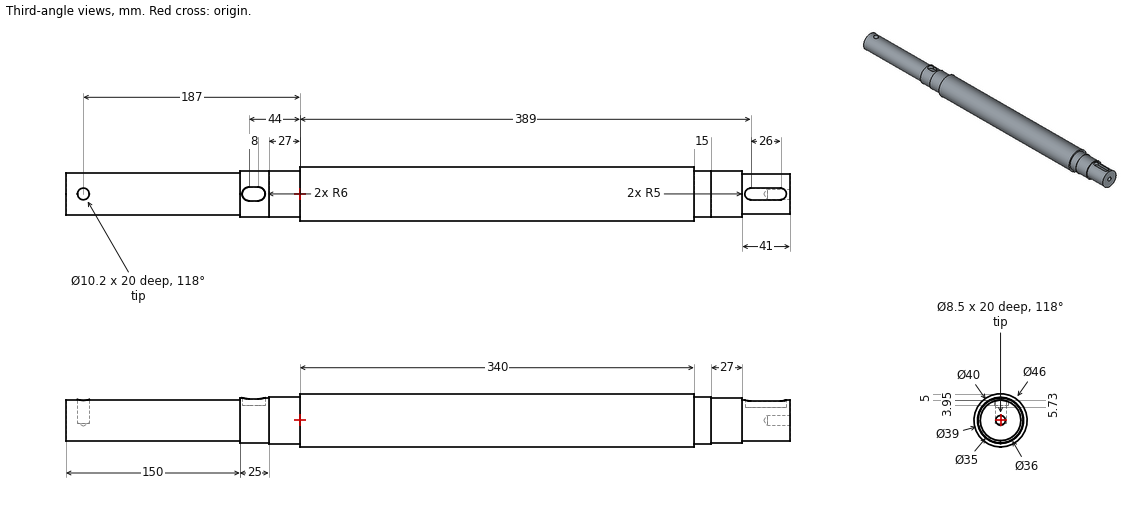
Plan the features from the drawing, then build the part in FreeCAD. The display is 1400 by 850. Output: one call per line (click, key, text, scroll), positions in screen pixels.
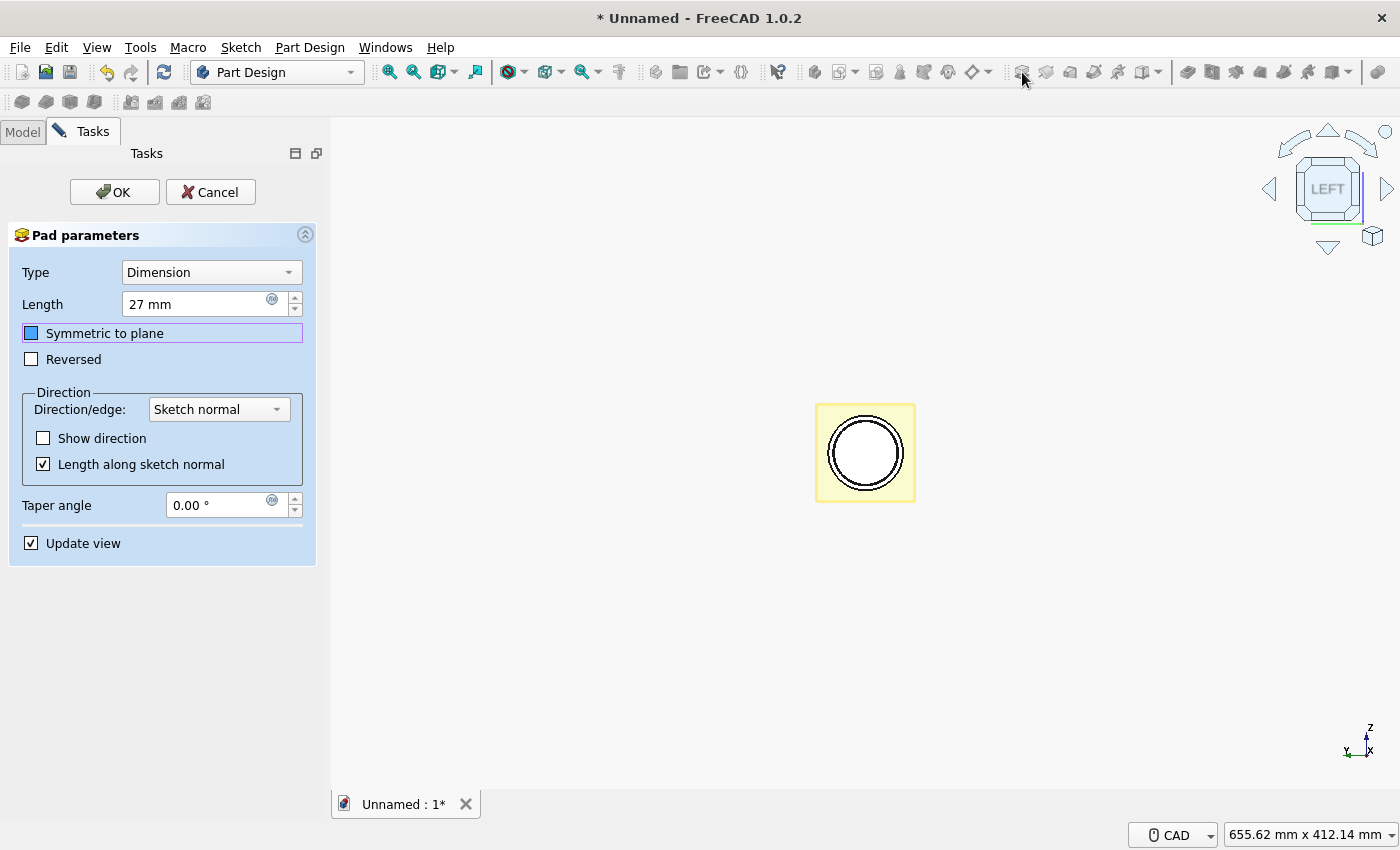
click(30, 359)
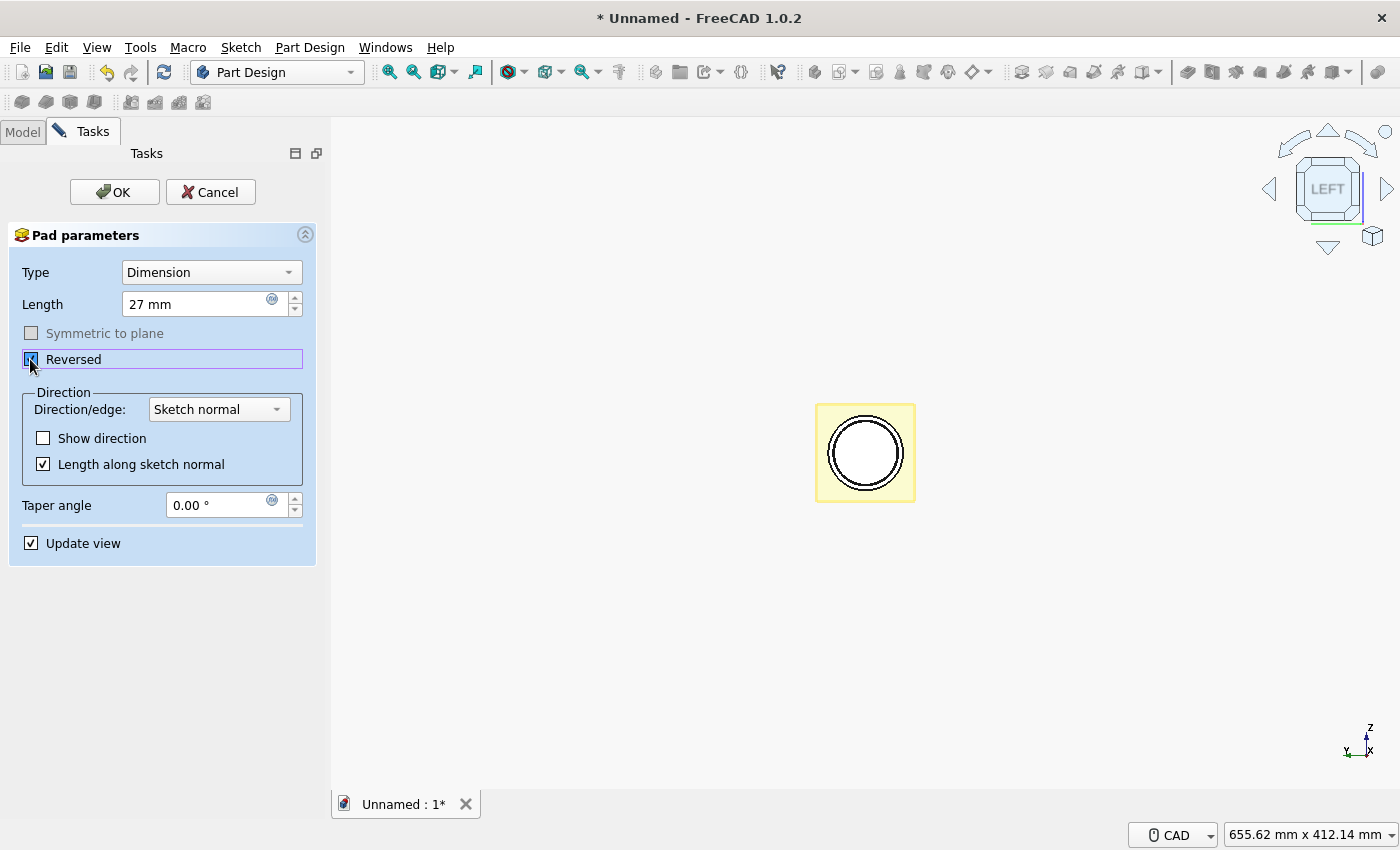
click(115, 192)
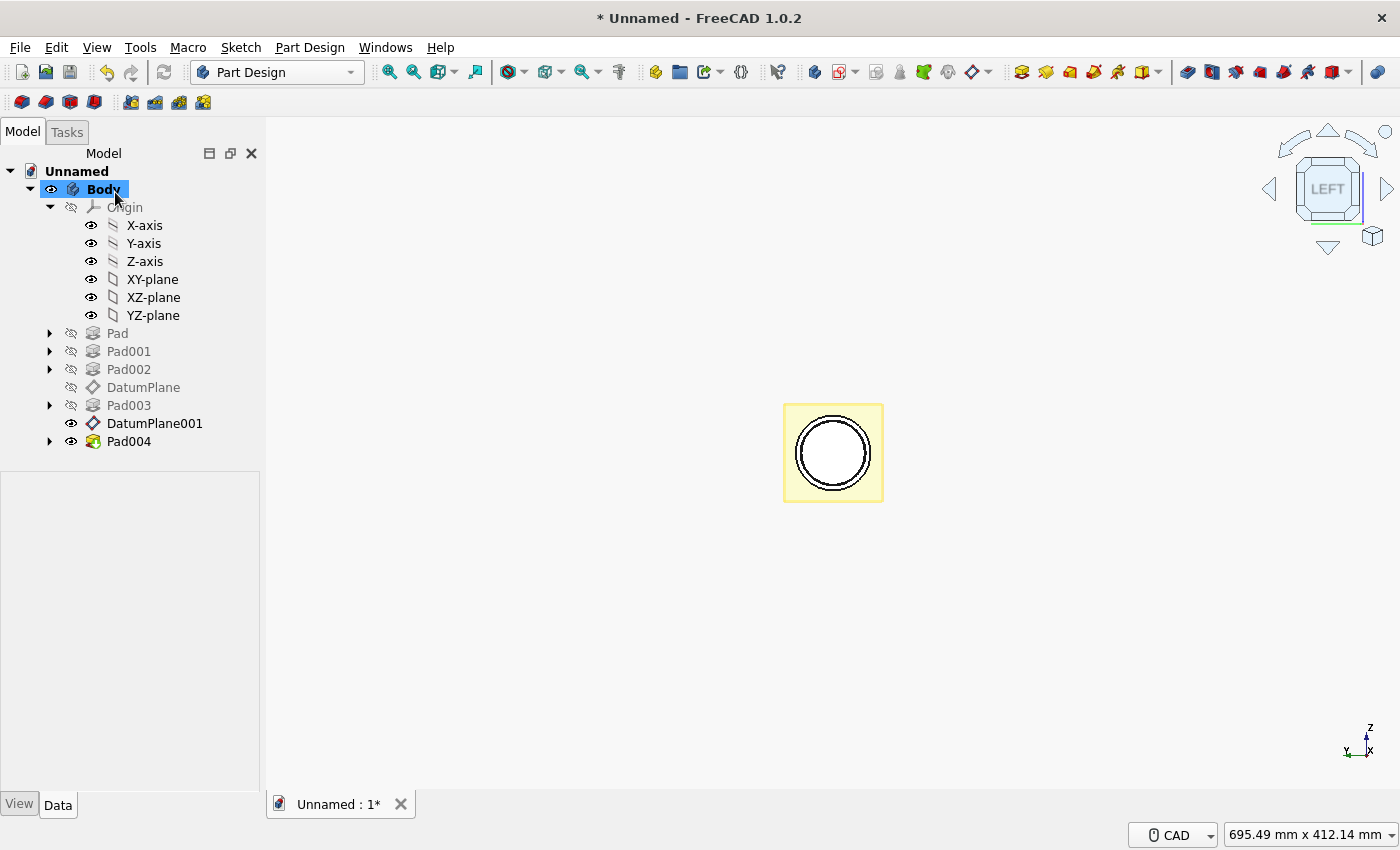
click(116, 423)
key(space)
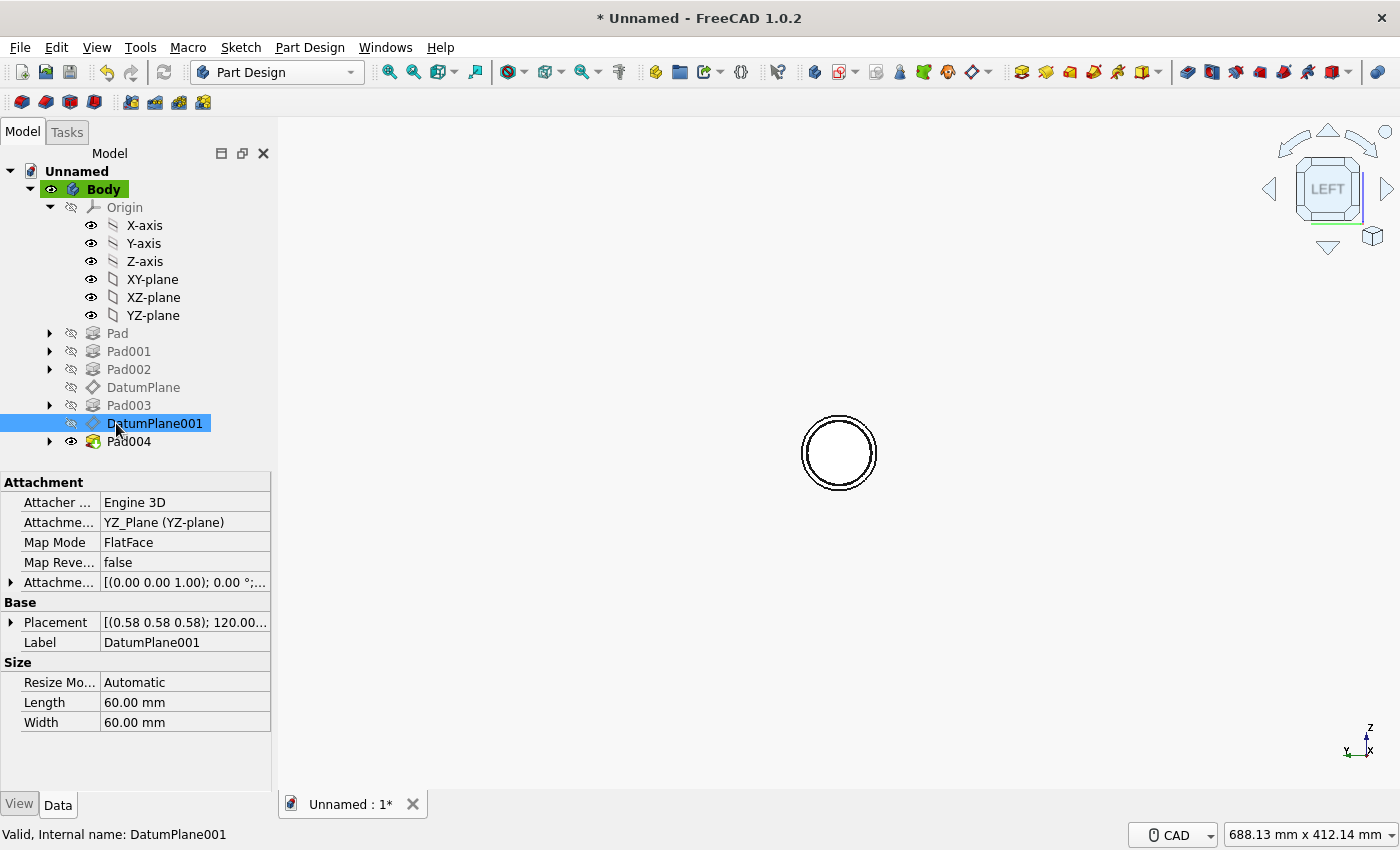
click(390, 72)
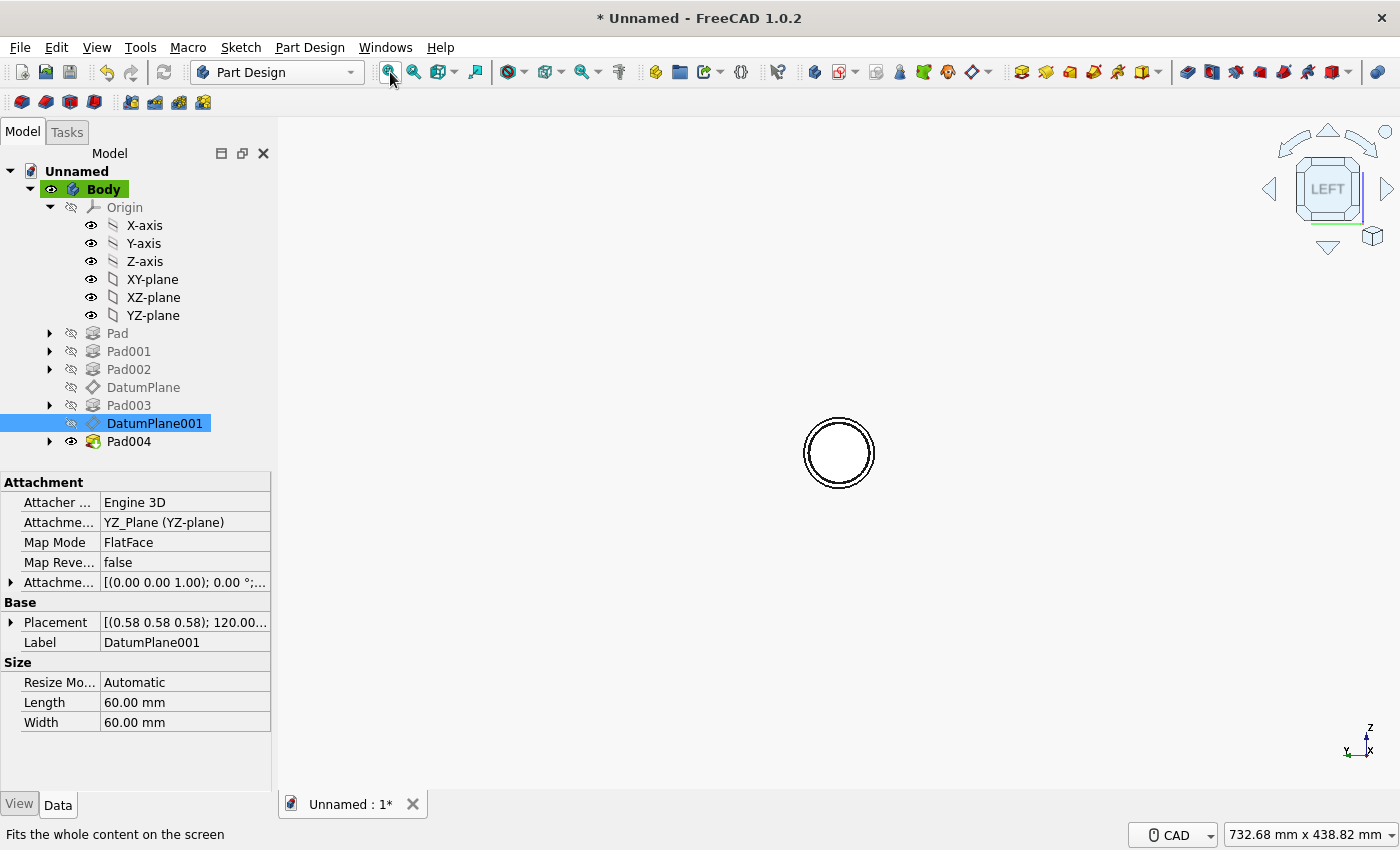
key(0)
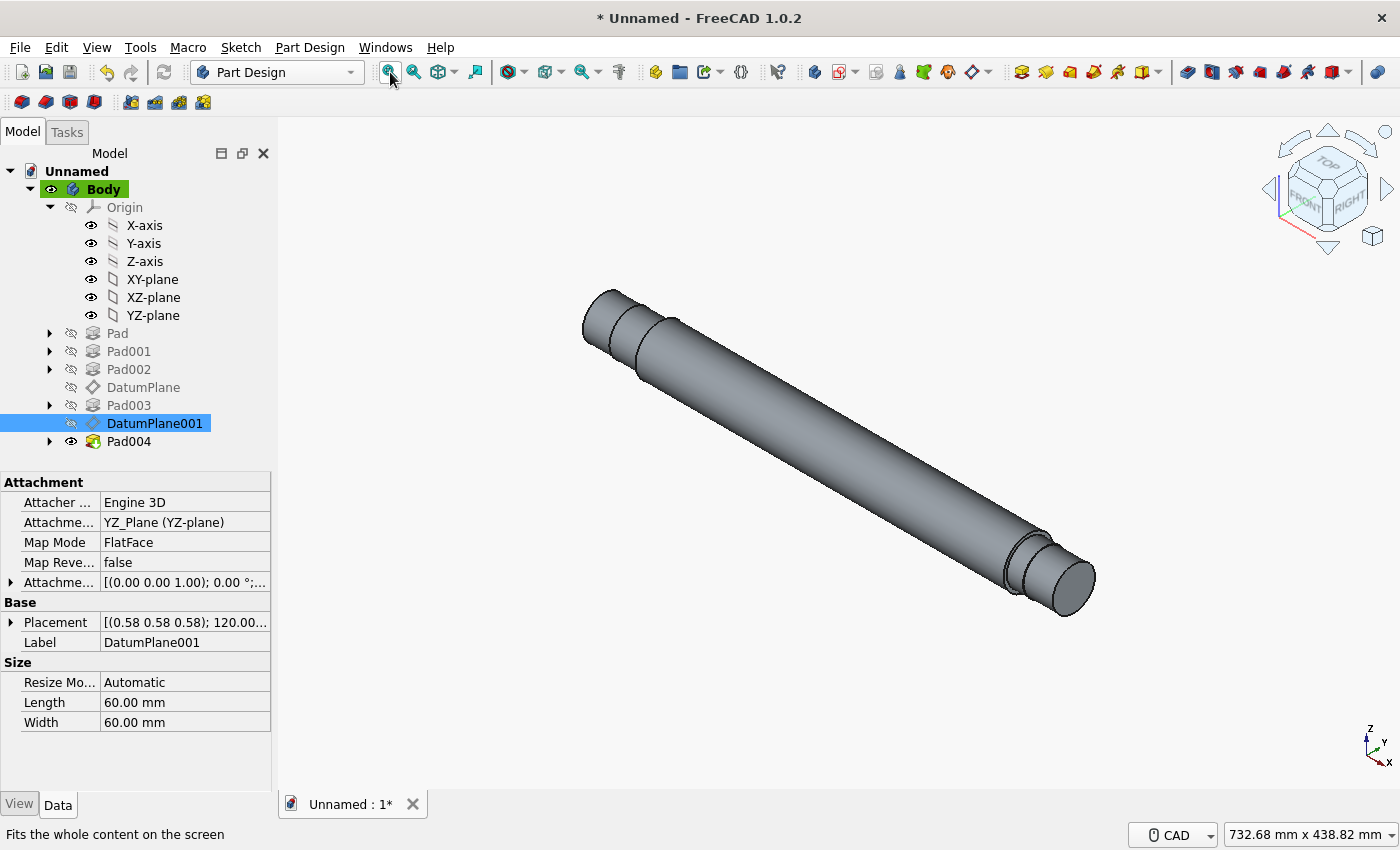
click(1074, 588)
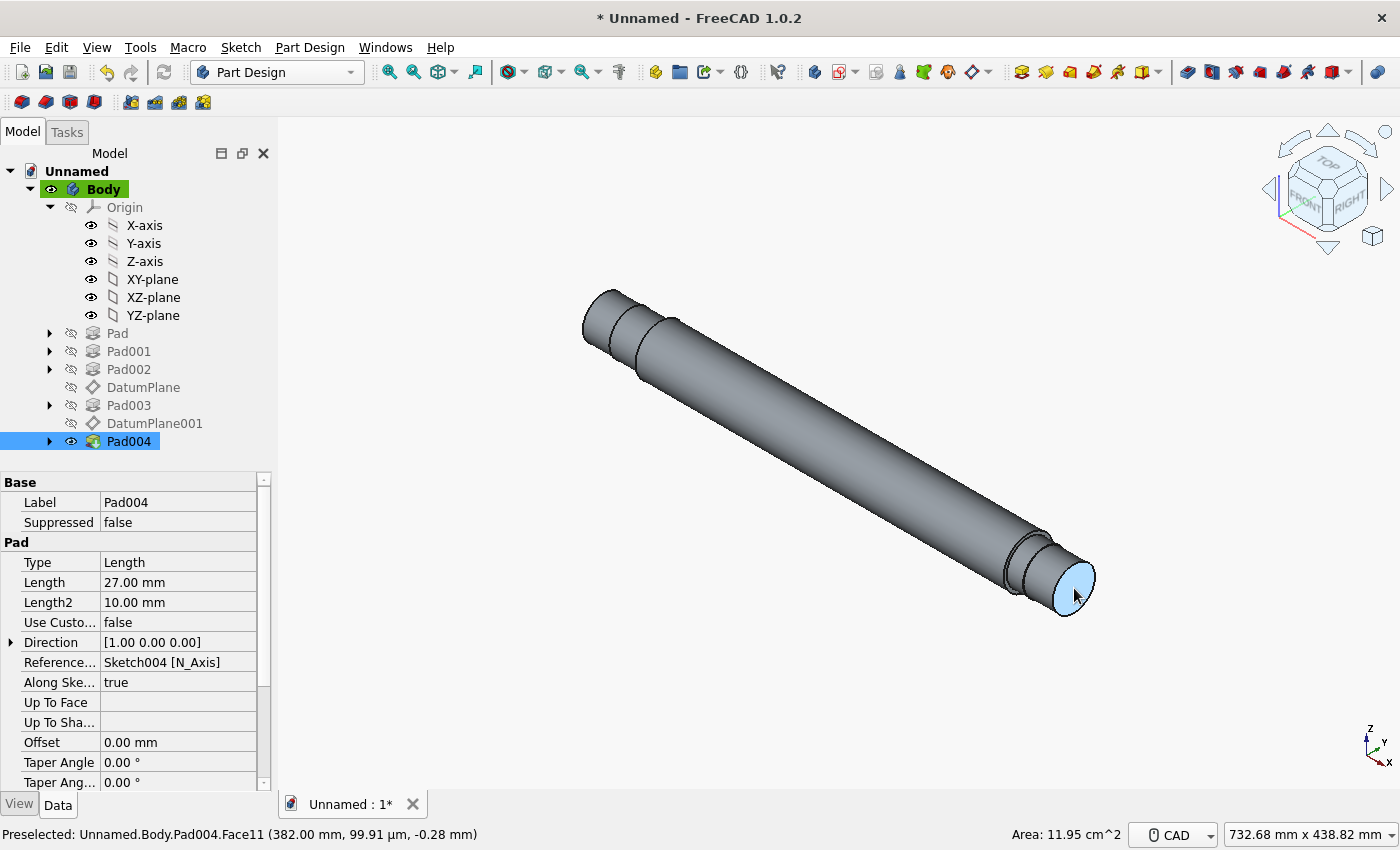
click(840, 72)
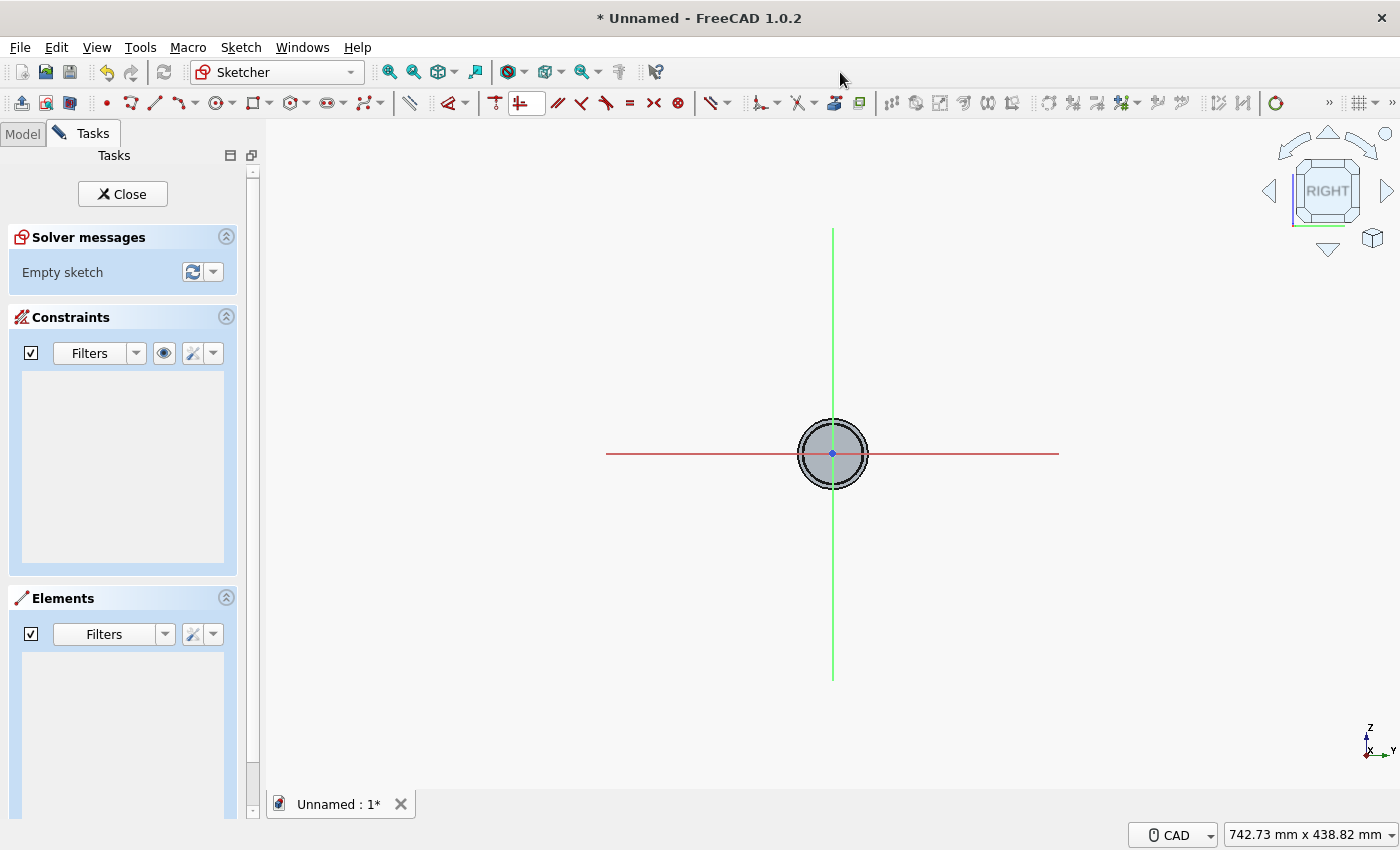
scroll(844, 454, up, 10)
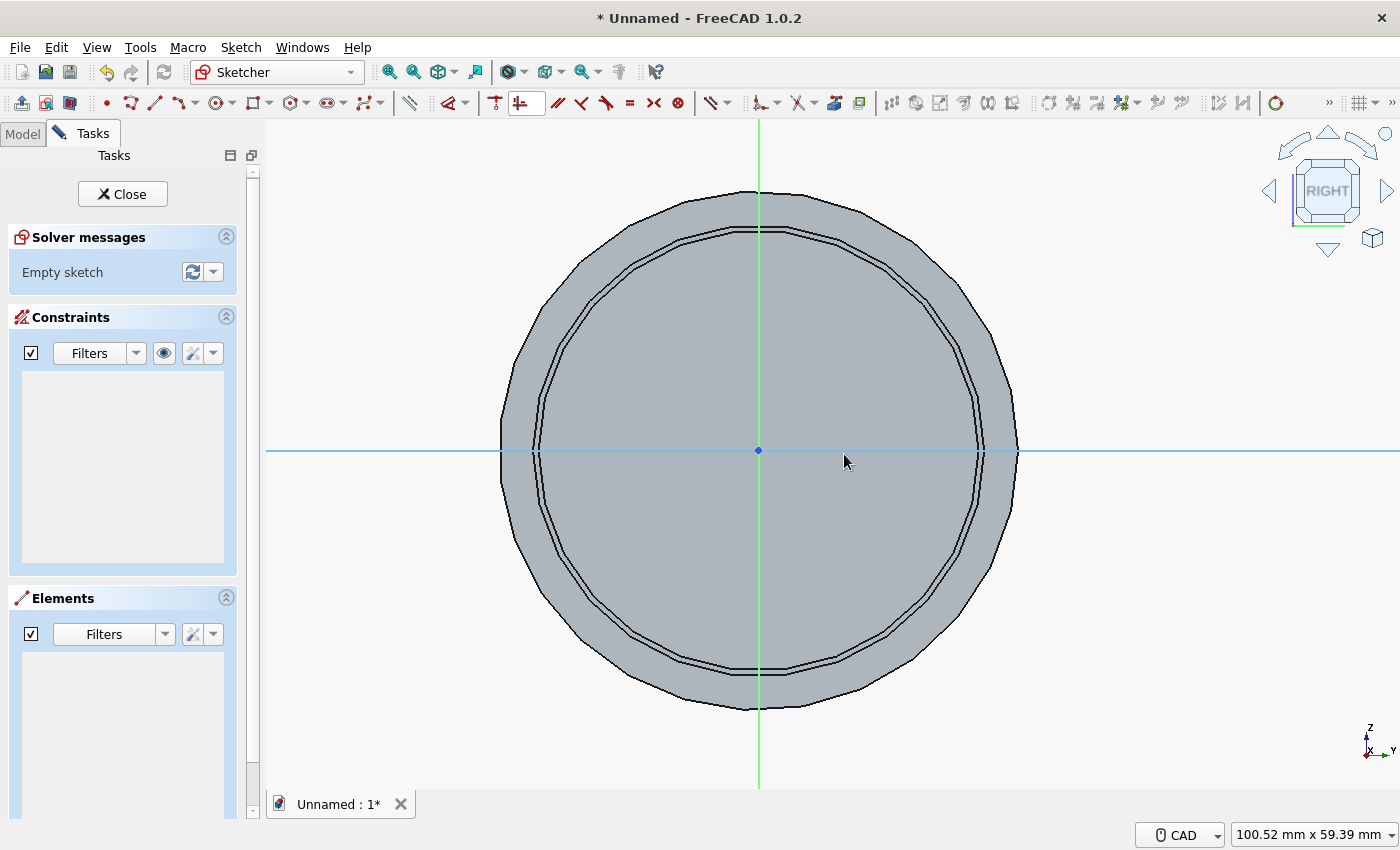
click(216, 104)